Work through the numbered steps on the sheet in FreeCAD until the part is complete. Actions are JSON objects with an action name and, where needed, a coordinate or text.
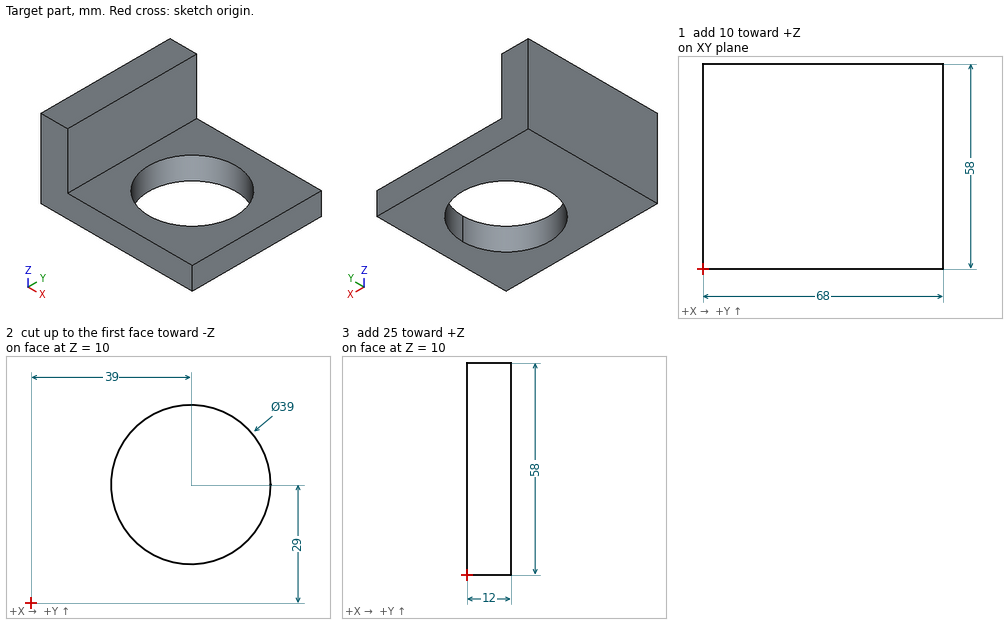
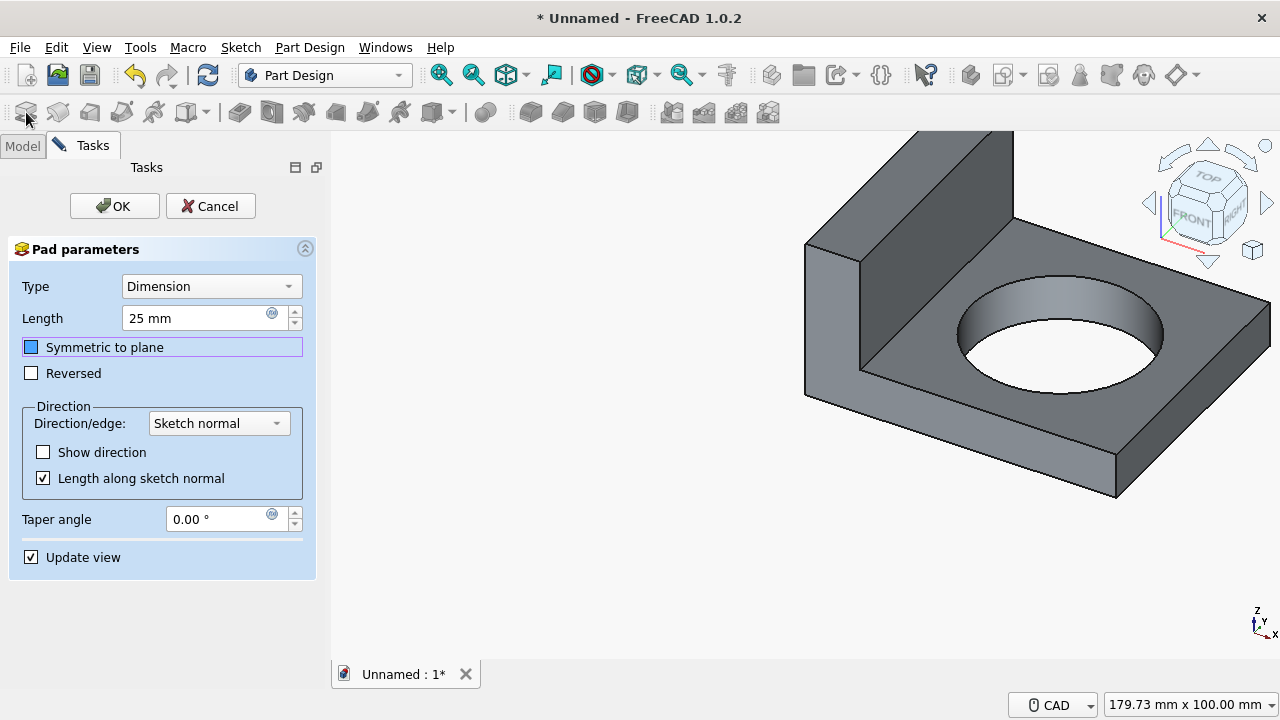
{"action": "left_click", "coordinate": [115, 206]}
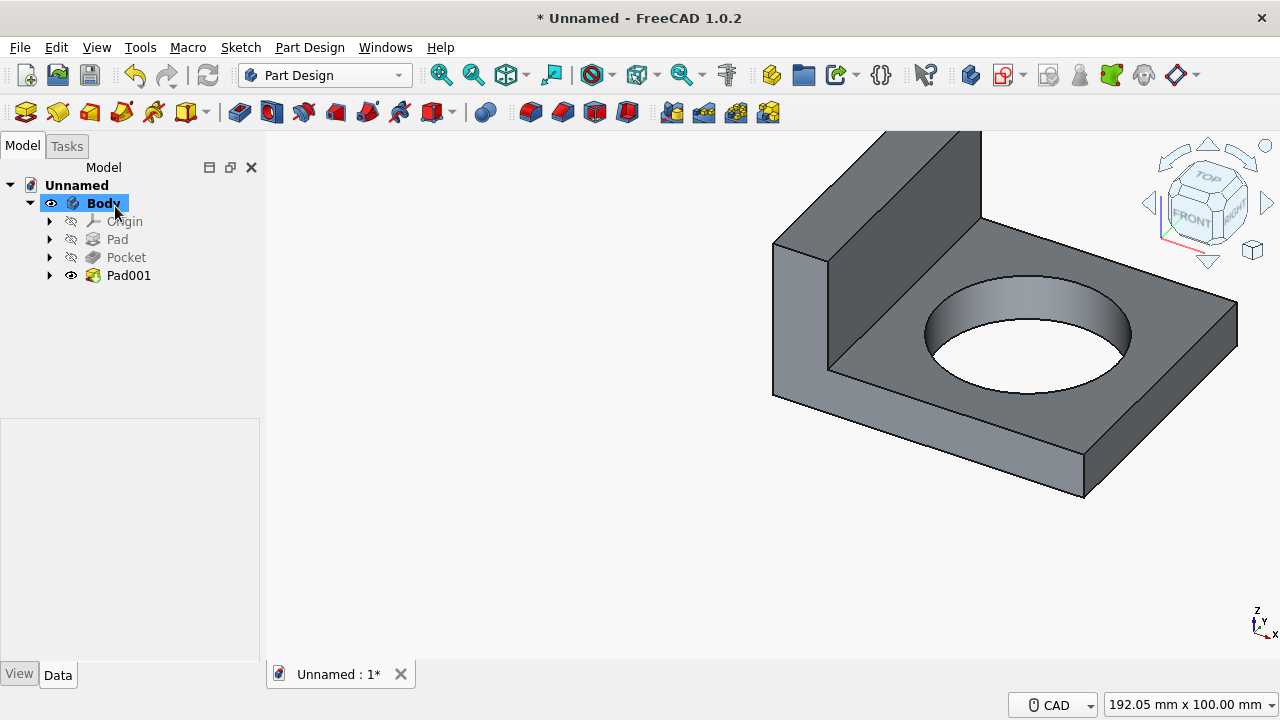
{"action": "key", "text": "0"}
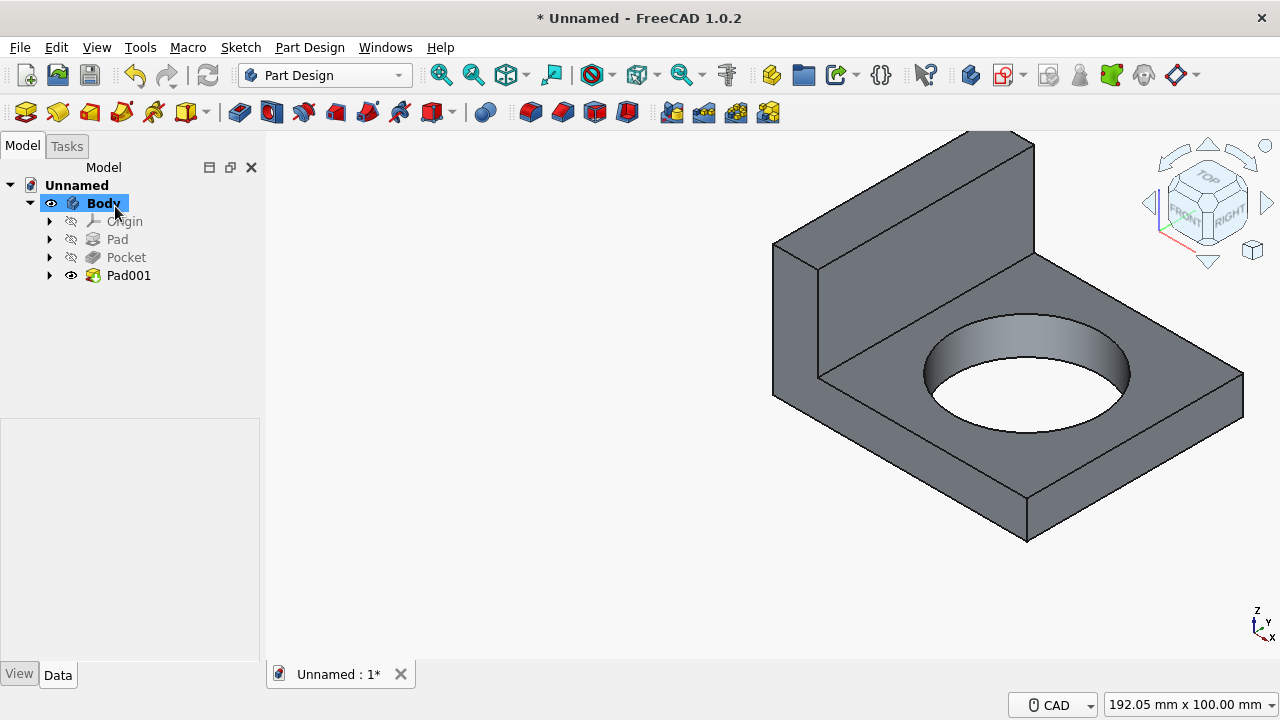
{"action": "key", "text": "v f"}